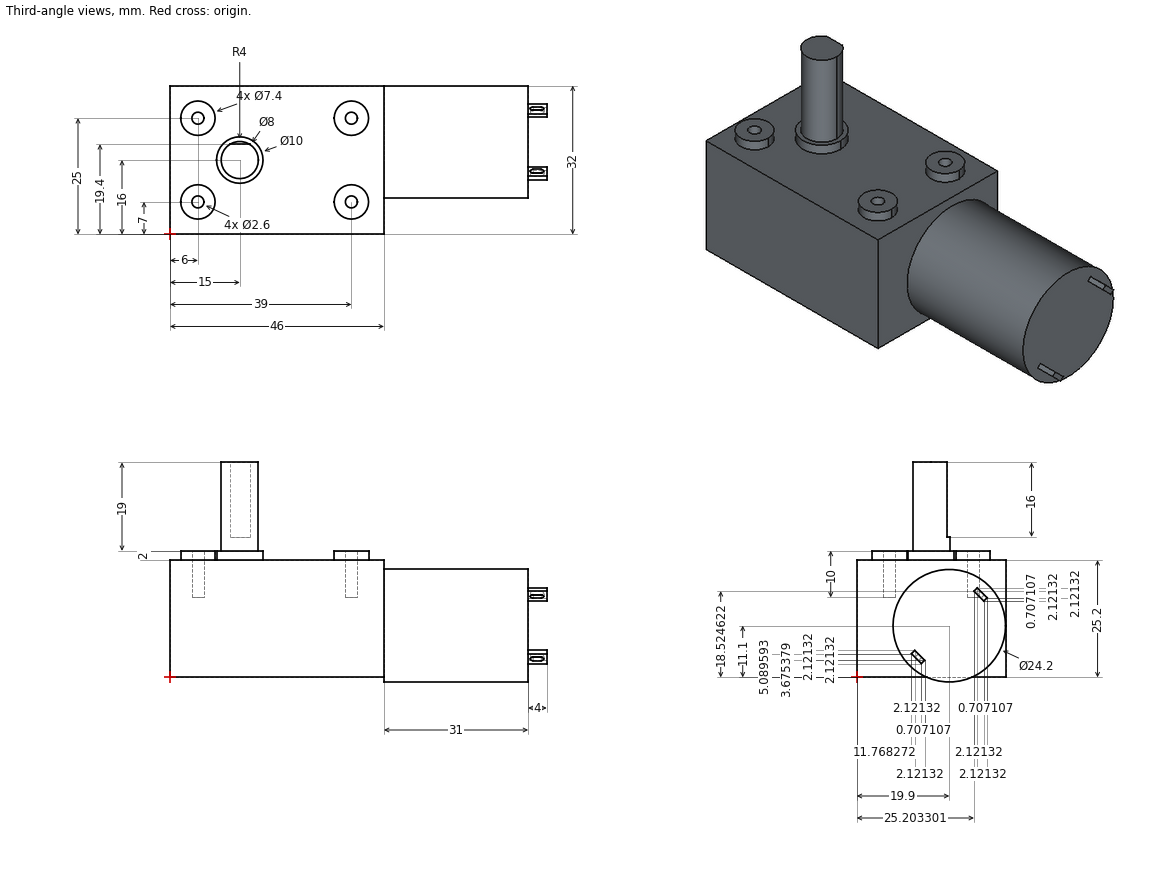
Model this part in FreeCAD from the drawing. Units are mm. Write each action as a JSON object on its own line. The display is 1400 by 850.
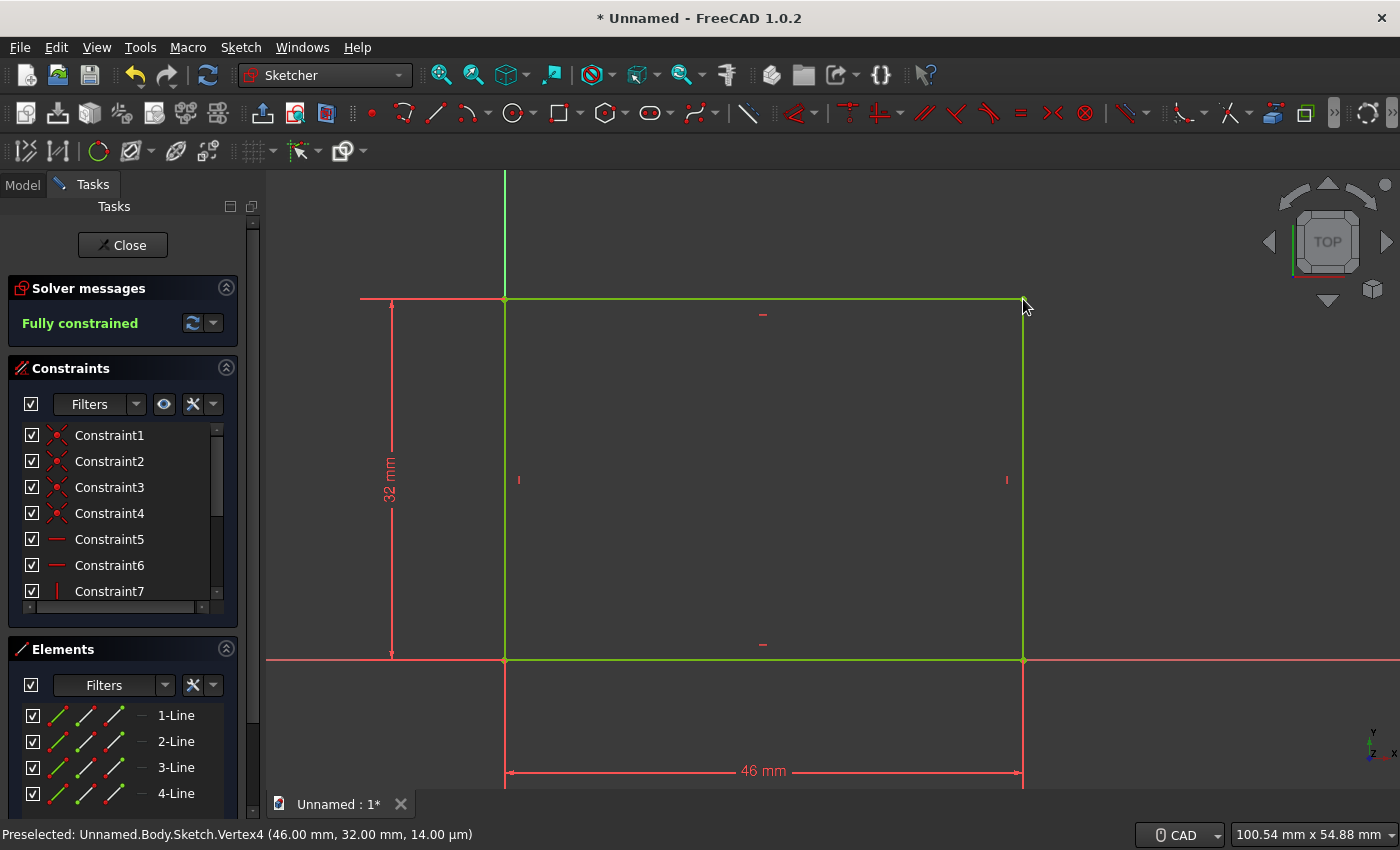
{"action": "left_click", "coordinate": [123, 245]}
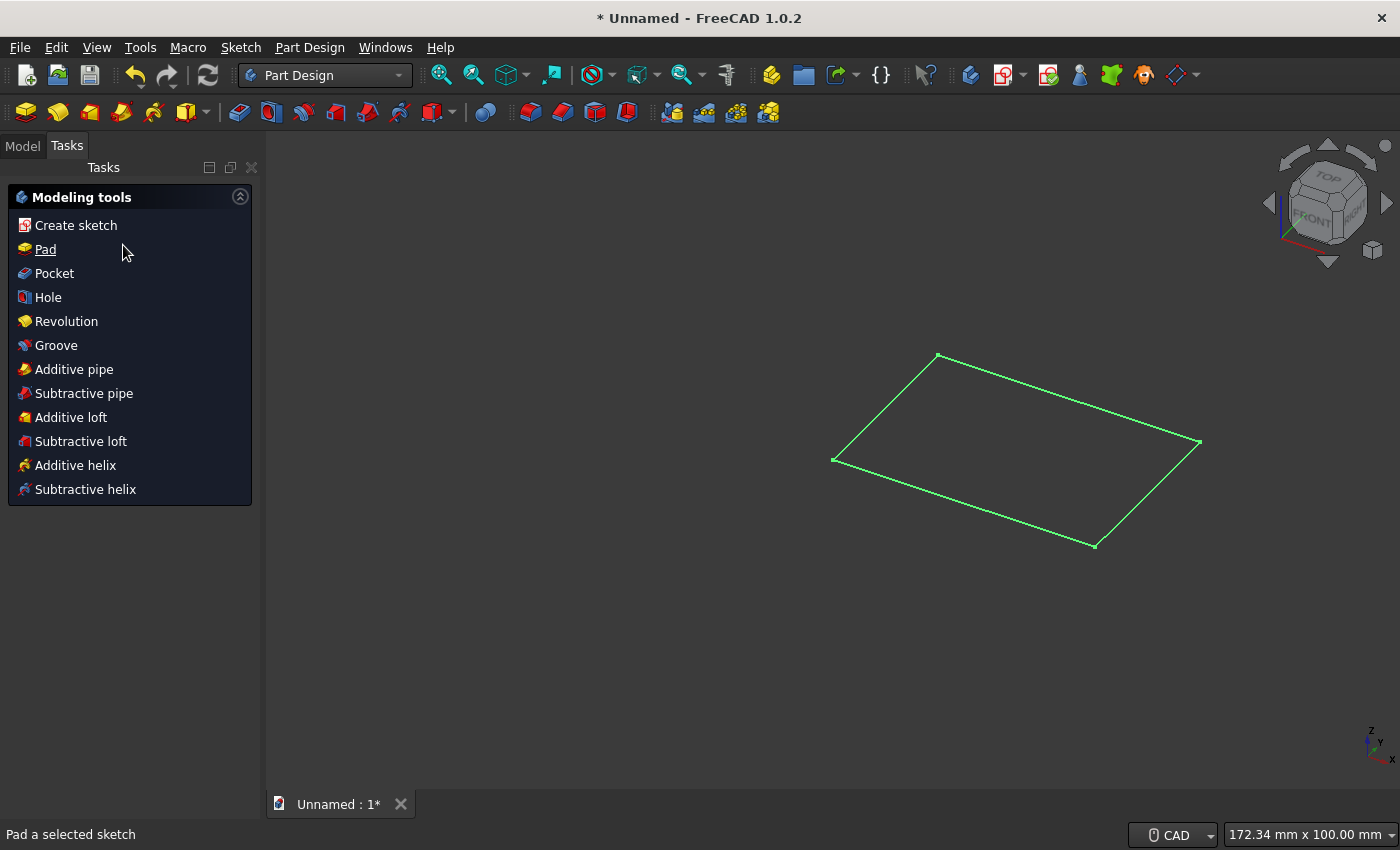
{"action": "left_click", "coordinate": [26, 112]}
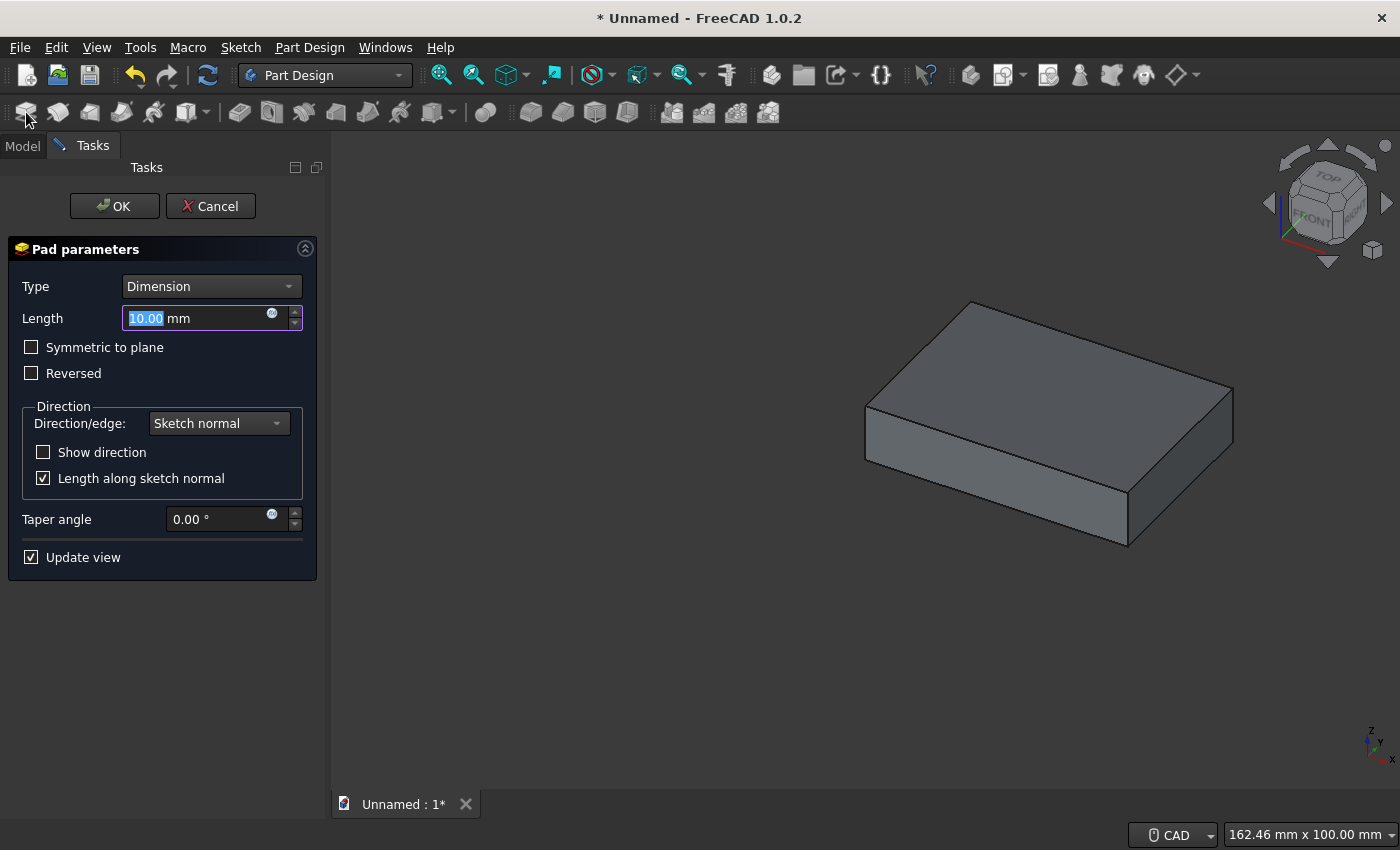
{"action": "type", "text": "25.2"}
{"action": "key", "text": "Tab"}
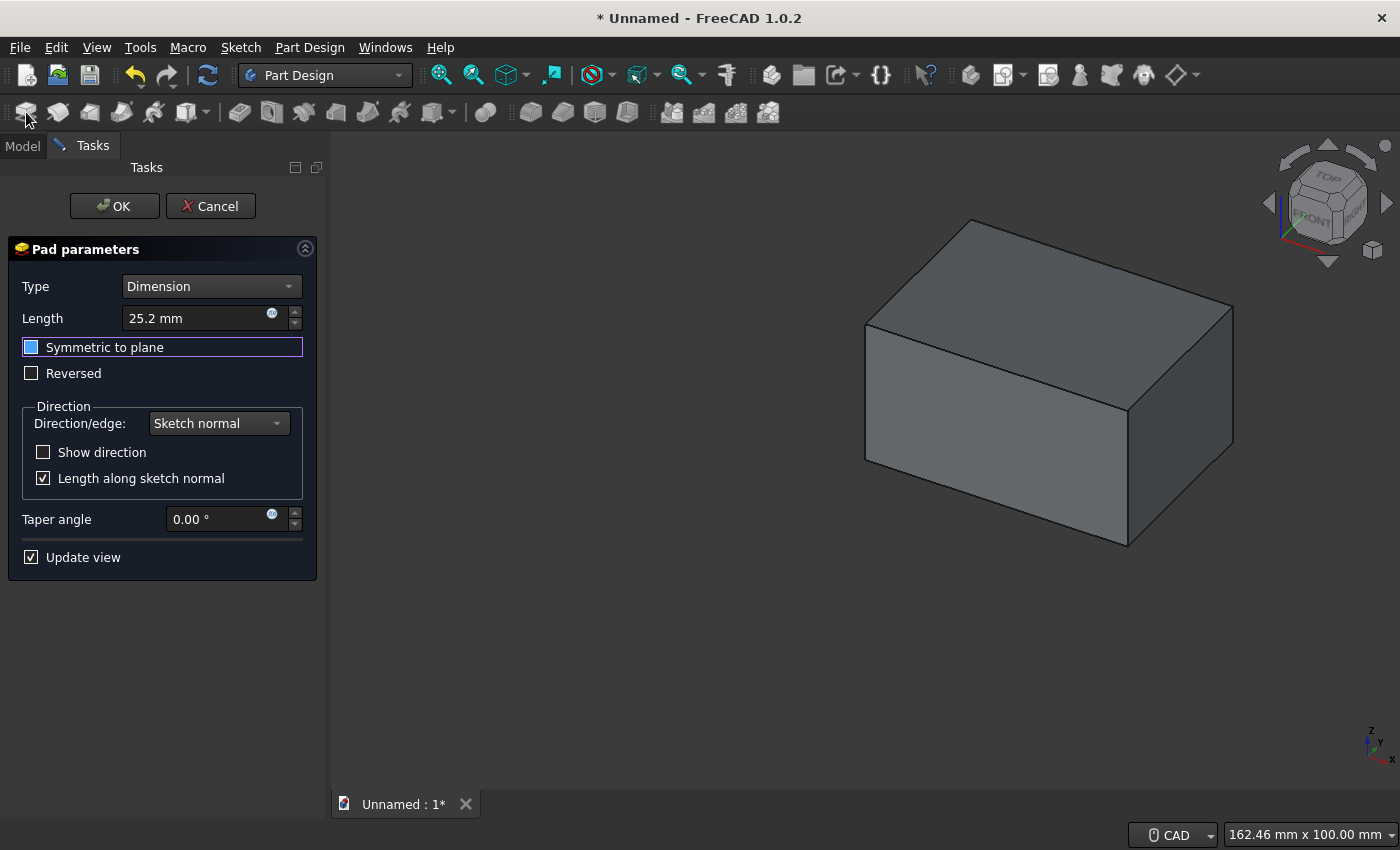
{"action": "left_click", "coordinate": [115, 206]}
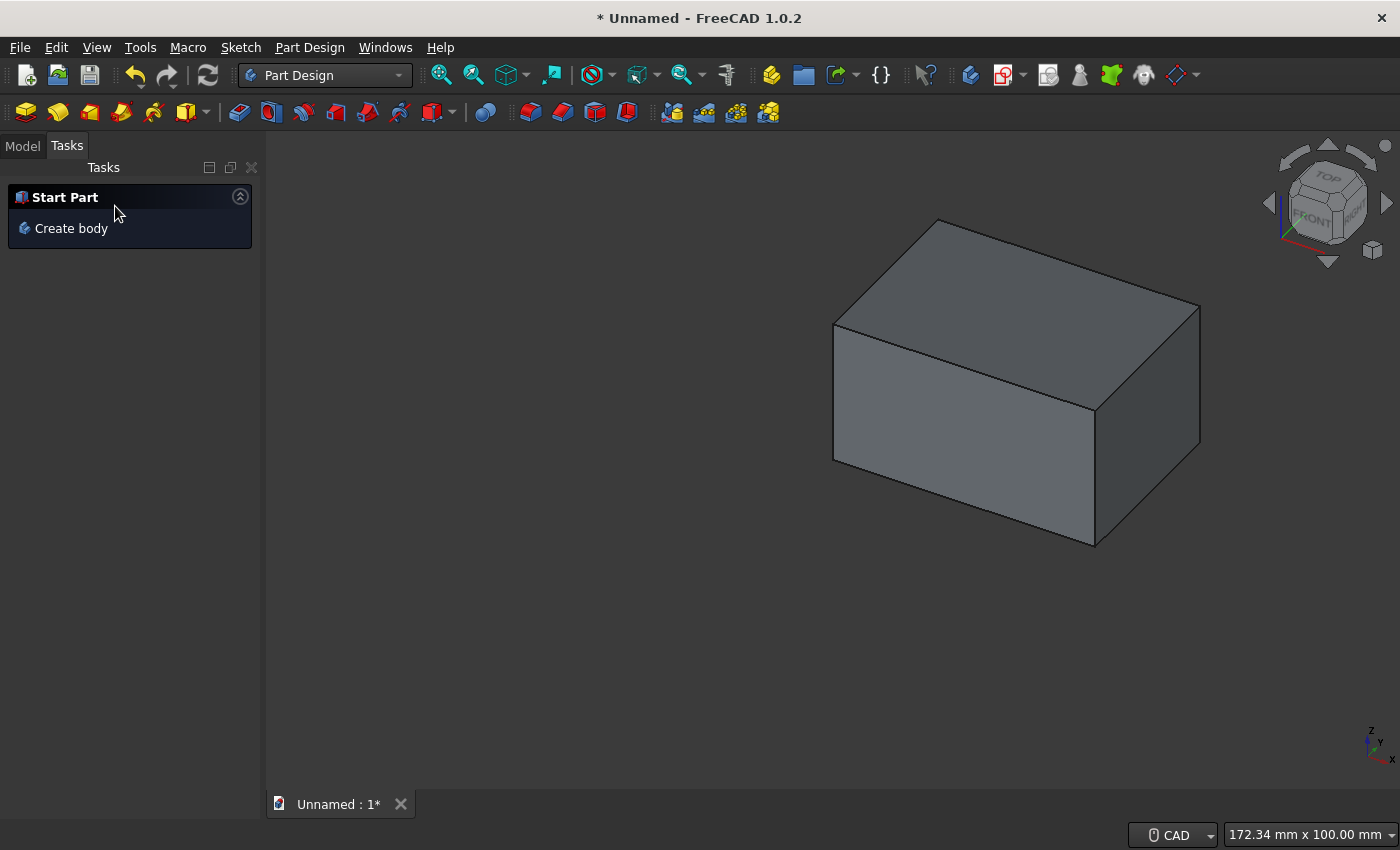
{"action": "left_click", "coordinate": [1054, 327]}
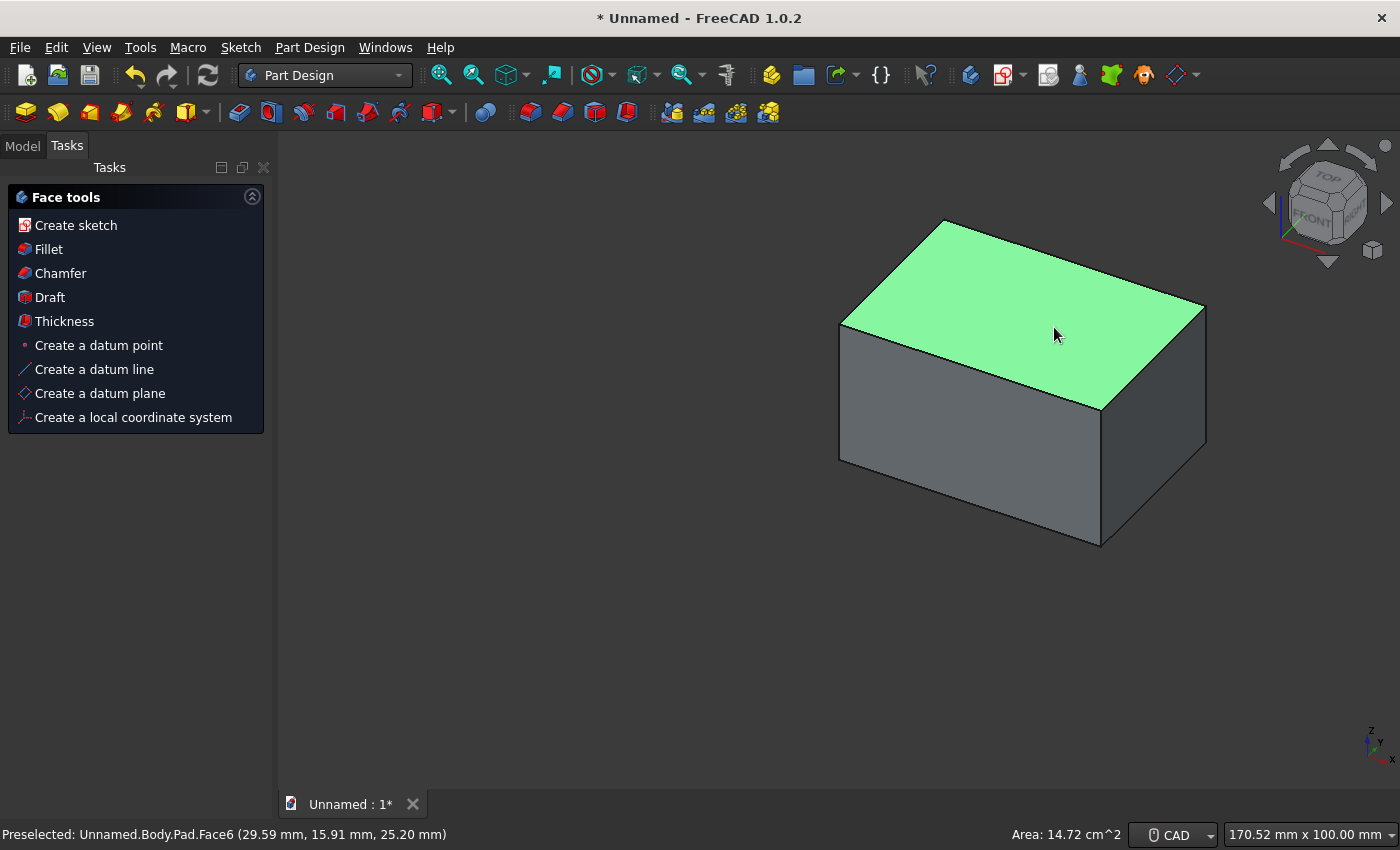
{"action": "left_click", "coordinate": [1004, 76]}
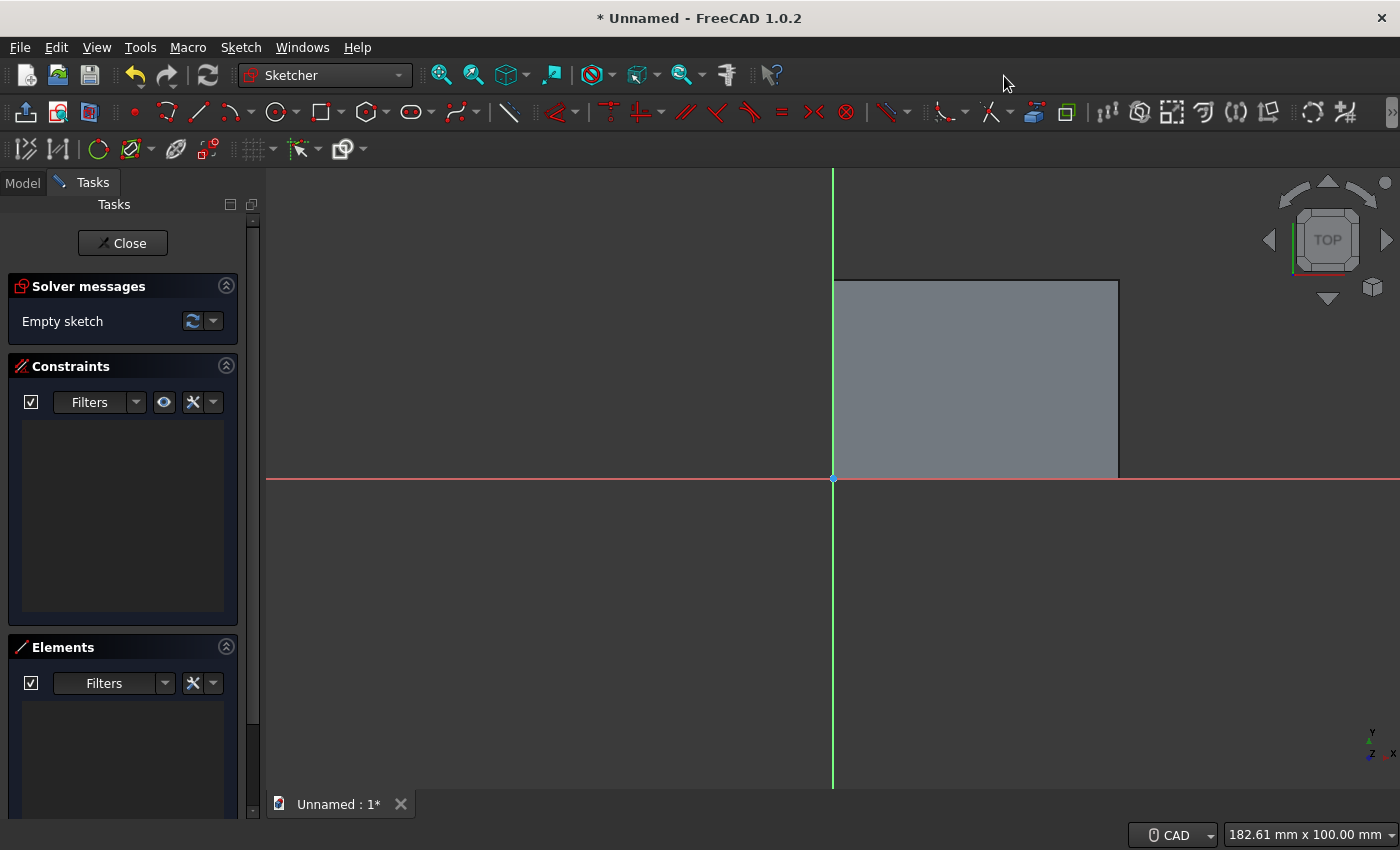
{"action": "scroll", "coordinate": [1130, 317], "scroll_direction": "up", "scroll_amount": 4}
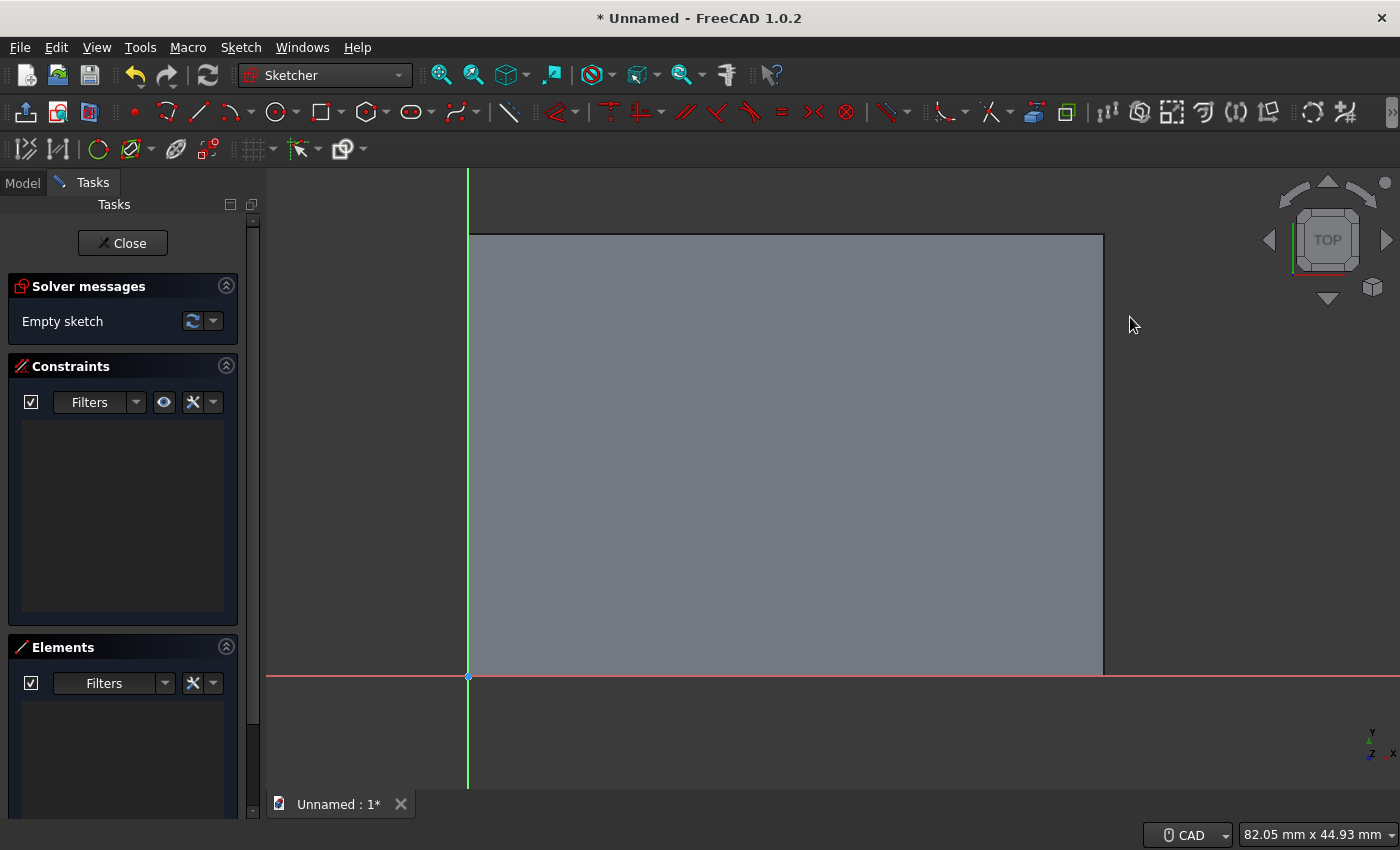
{"action": "left_click", "coordinate": [276, 112]}